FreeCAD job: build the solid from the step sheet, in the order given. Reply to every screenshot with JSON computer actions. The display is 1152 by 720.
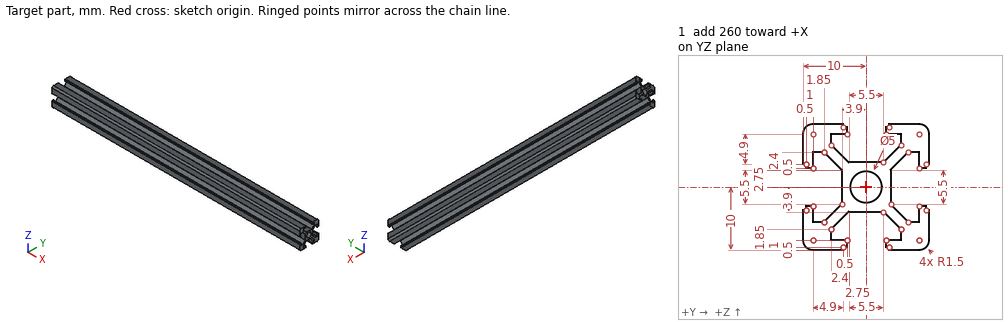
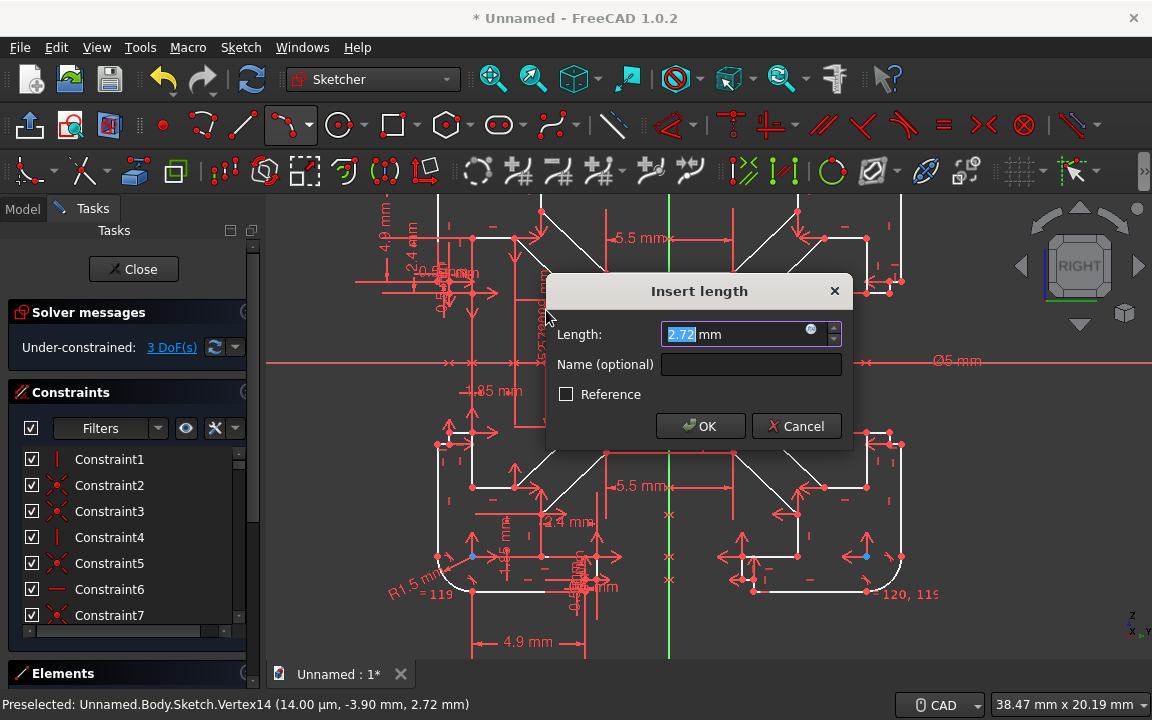
{"action": "type", "text": "2.75"}
{"action": "key", "text": "Return"}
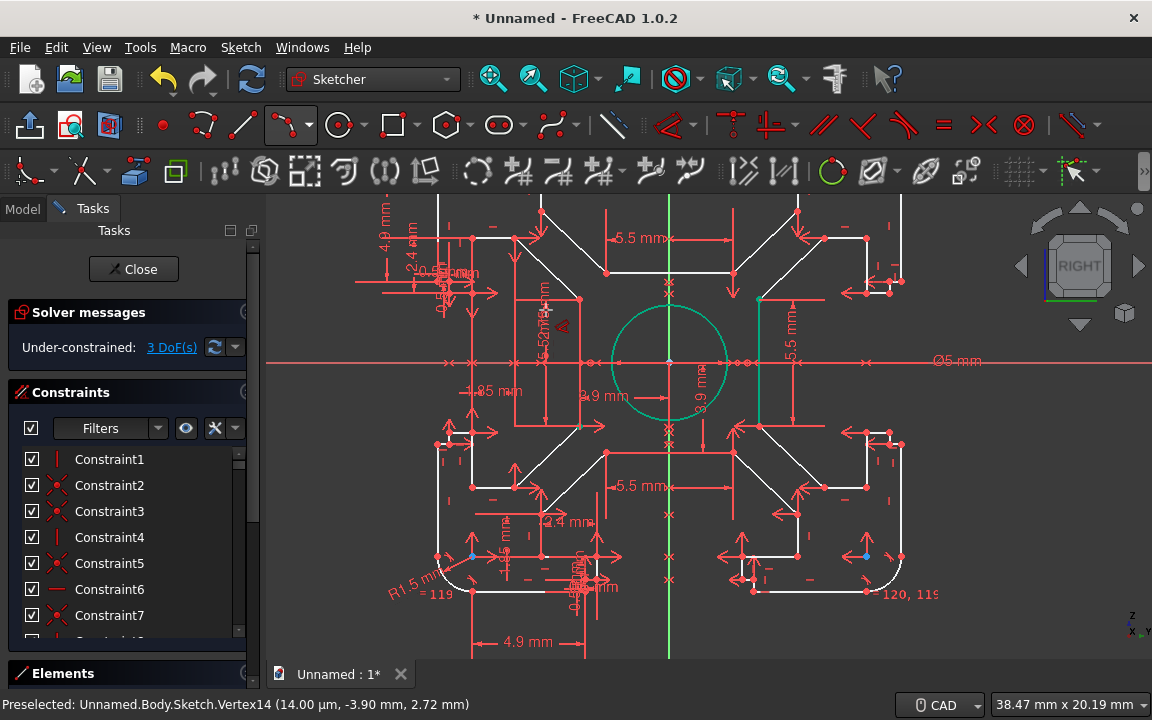
{"action": "left_click", "coordinate": [606, 453]}
{"action": "left_click", "coordinate": [652, 329]}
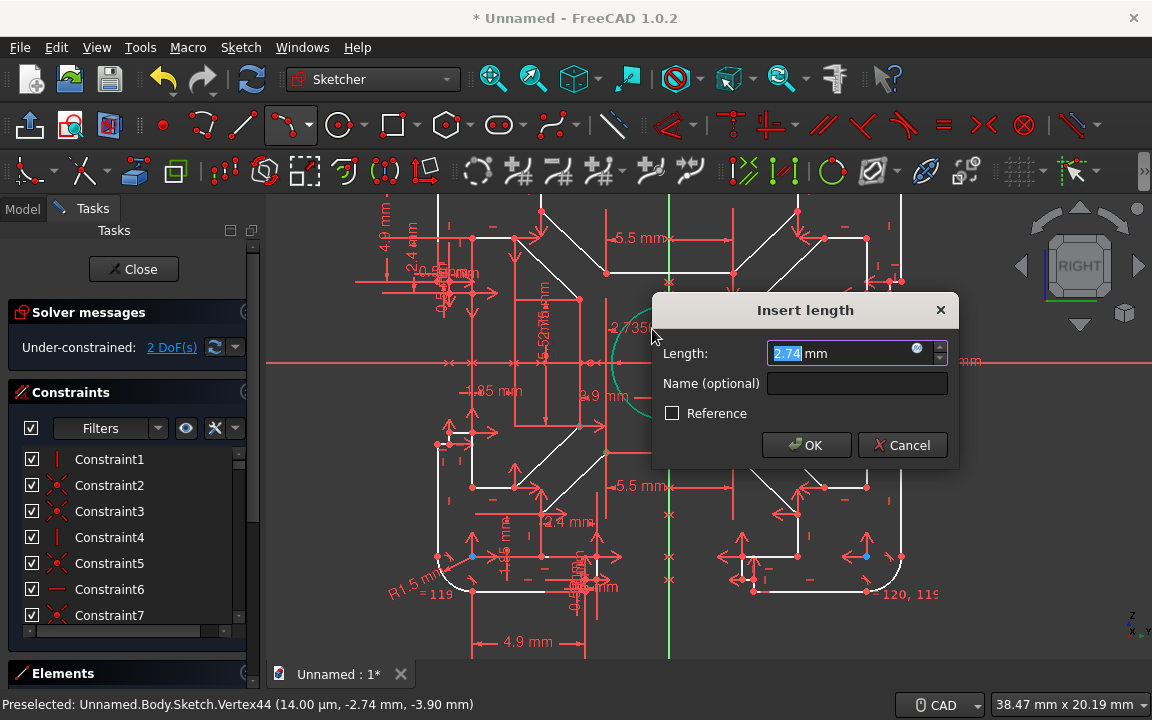
{"action": "type", "text": "2.75"}
{"action": "key", "text": "Return"}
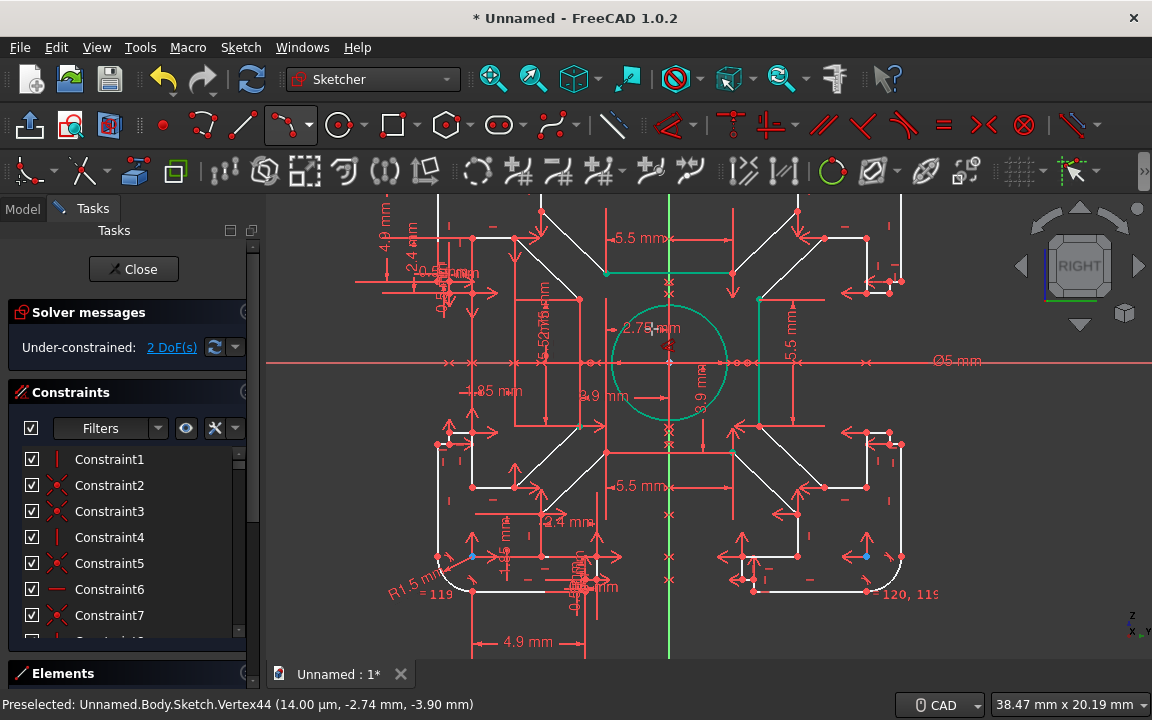
{"action": "scroll", "coordinate": [582, 556], "scroll_direction": "down", "scroll_amount": 2}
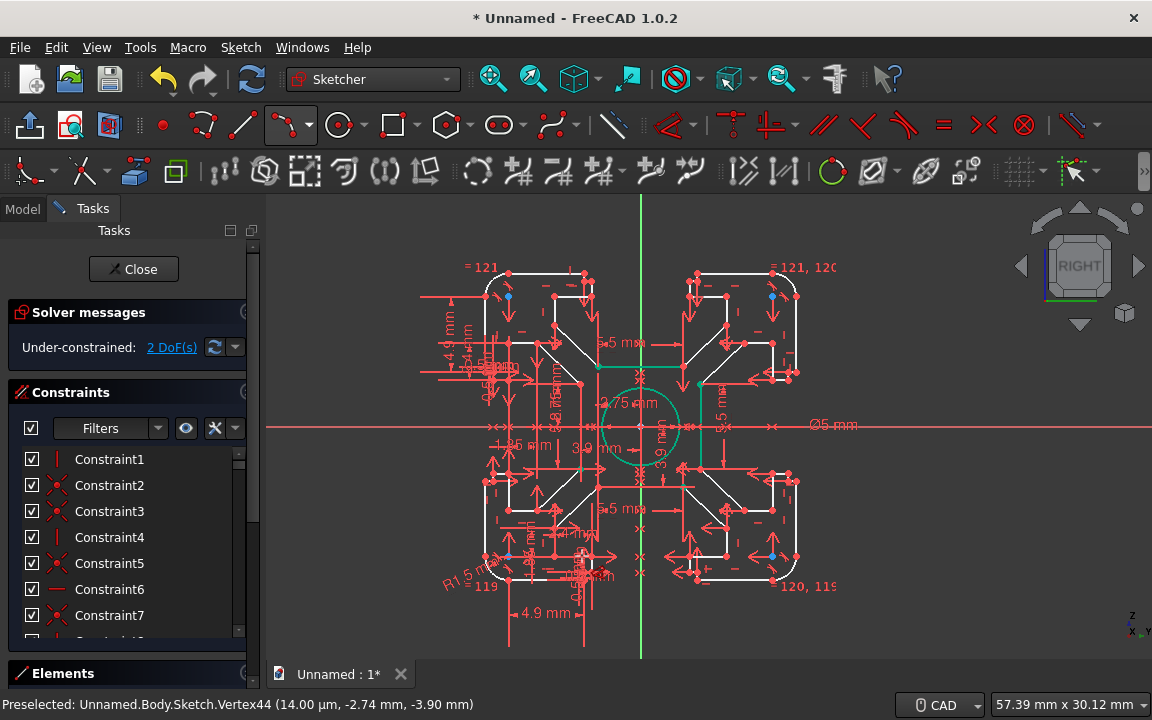
{"action": "left_click", "coordinate": [485, 297]}
{"action": "left_click", "coordinate": [599, 263]}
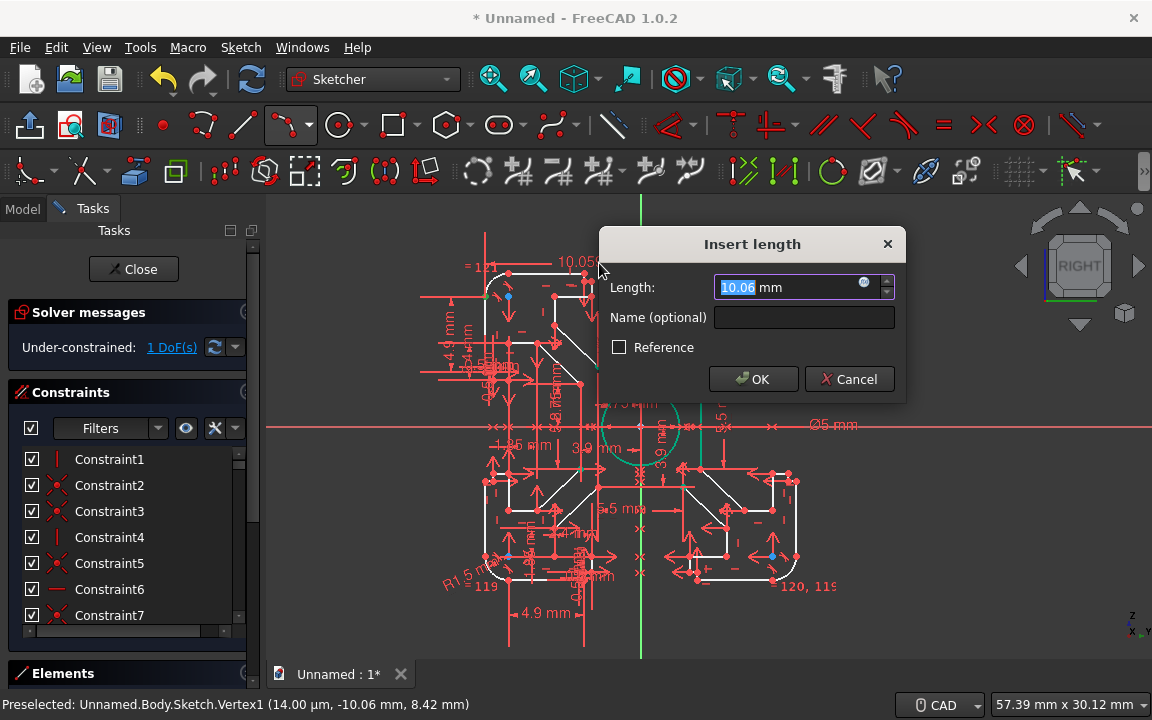
{"action": "type", "text": "10"}
{"action": "key", "text": "Return"}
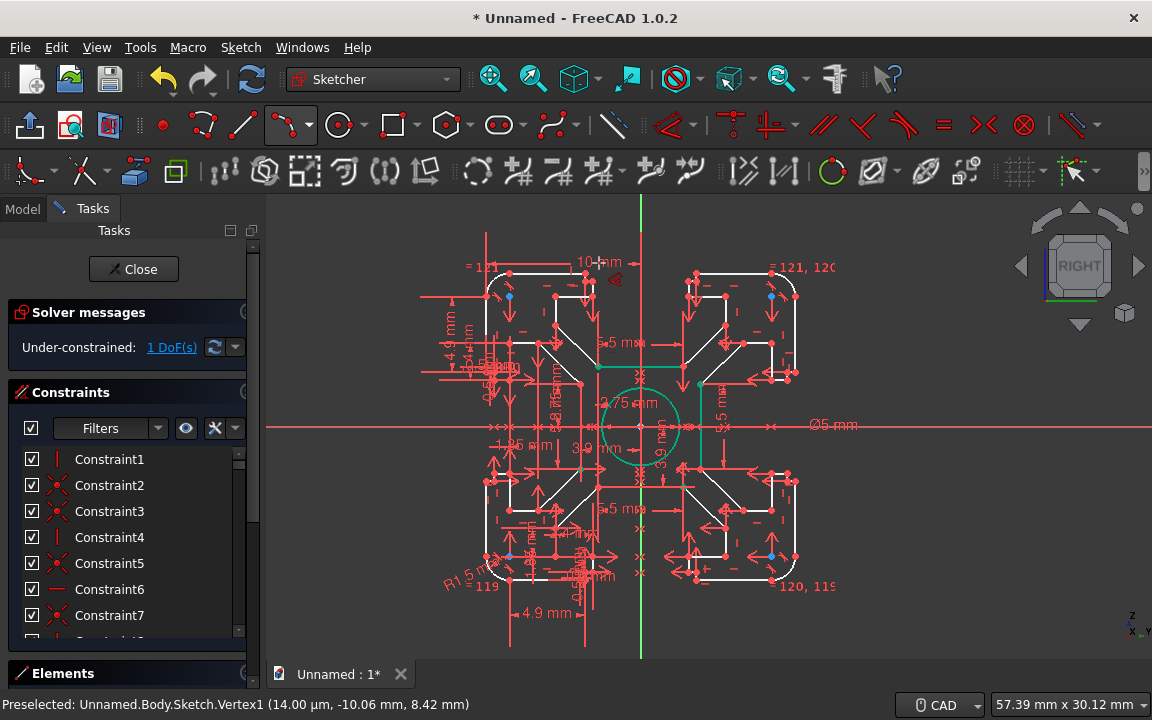
{"action": "left_click", "coordinate": [510, 580]}
{"action": "left_click", "coordinate": [476, 468]}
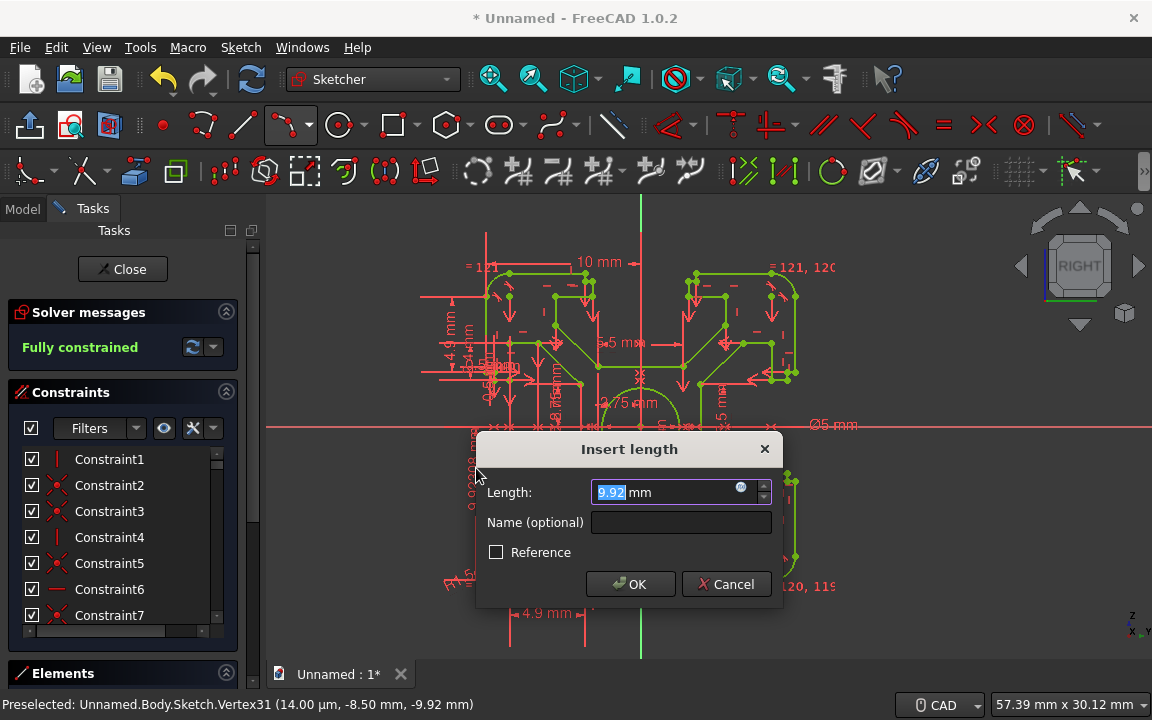
{"action": "type", "text": "10"}
{"action": "key", "text": "Return"}
{"action": "key", "text": "Escape"}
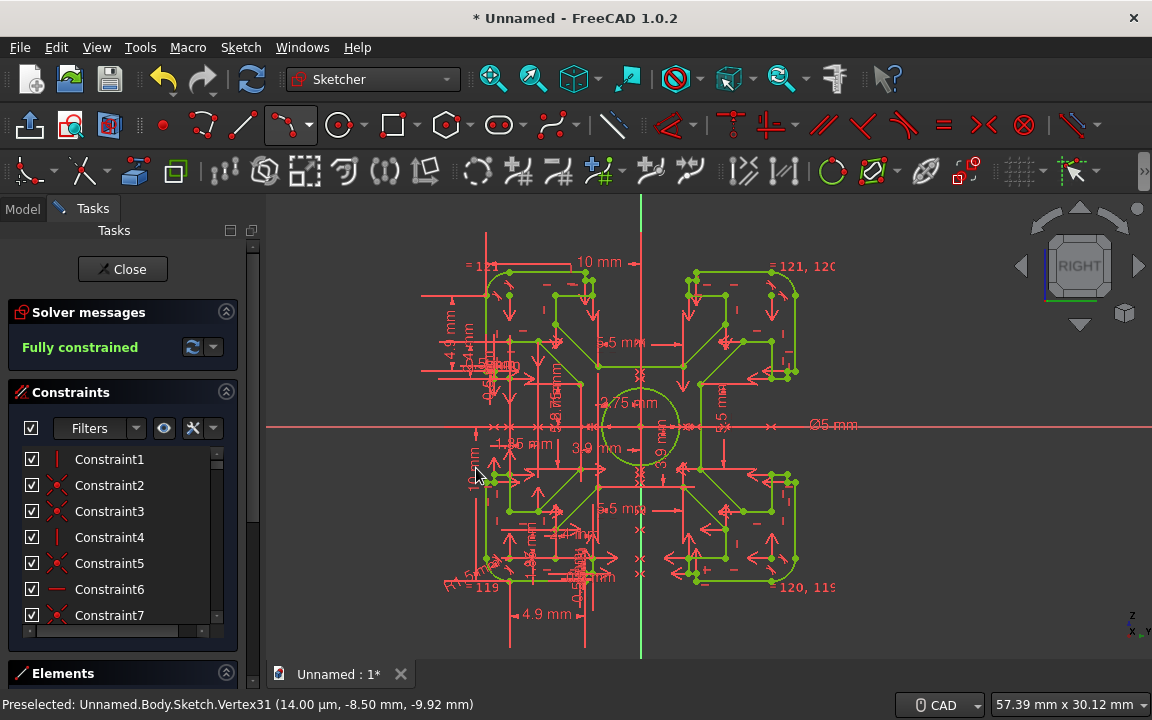
{"action": "left_click", "coordinate": [123, 269]}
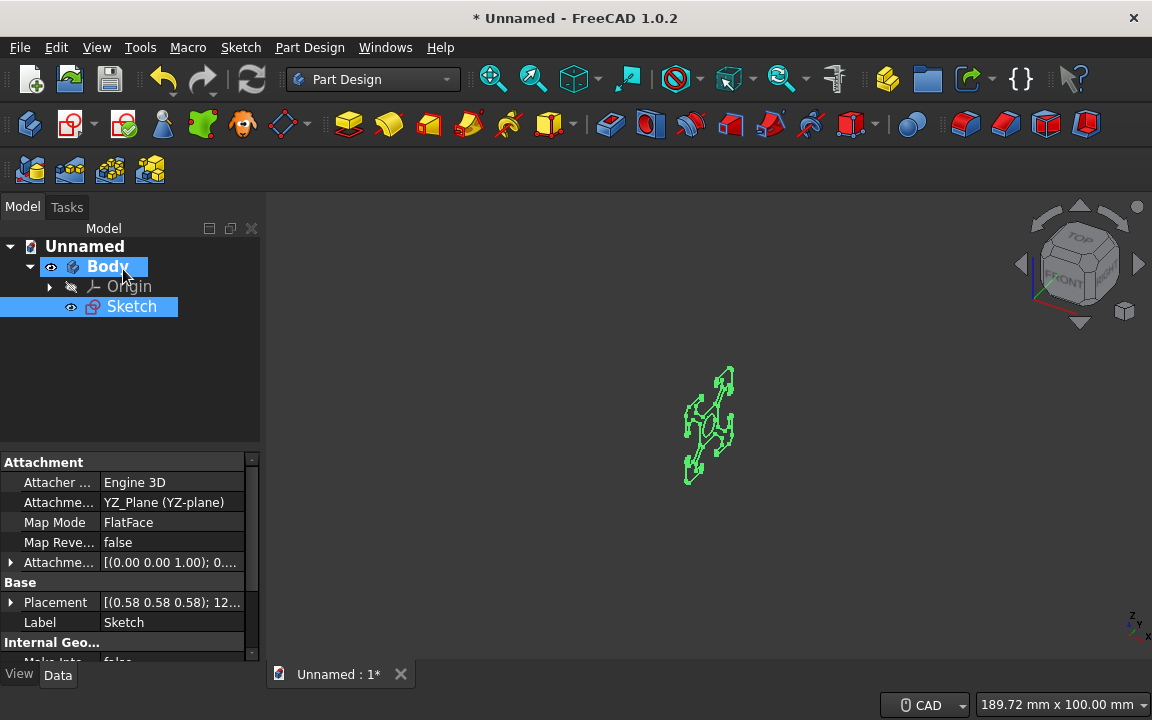
{"action": "left_click", "coordinate": [350, 124]}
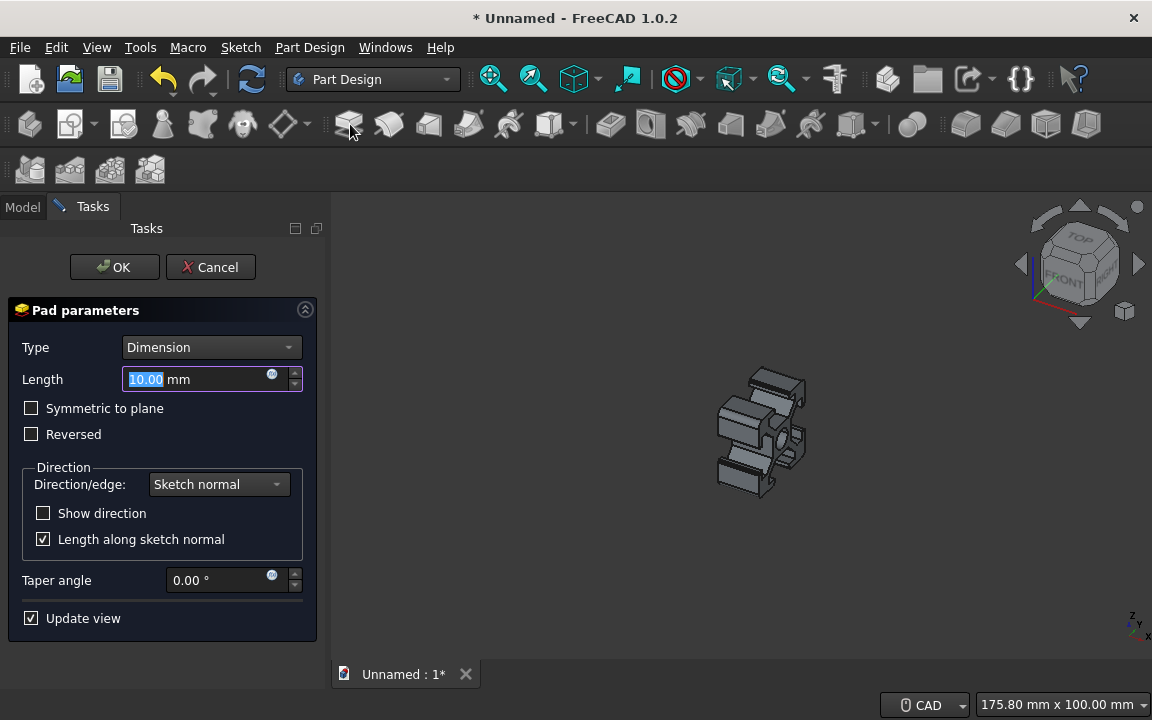
{"action": "type", "text": "260"}
{"action": "key", "text": "Tab"}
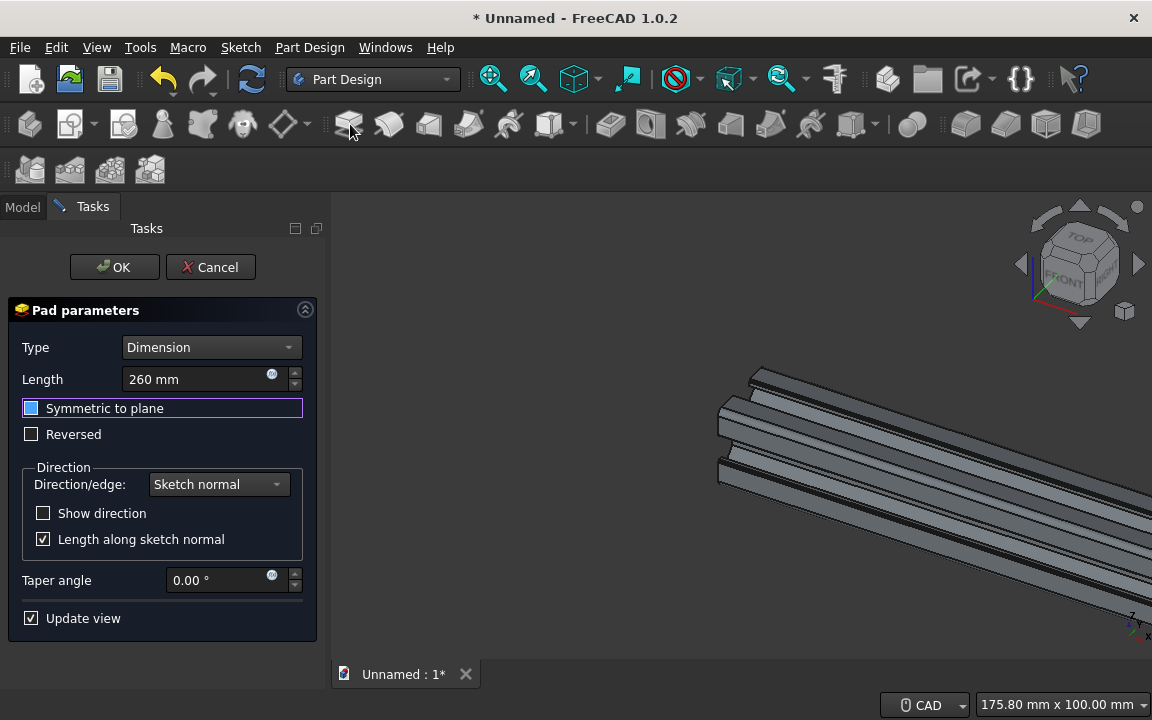
{"action": "left_click", "coordinate": [115, 267]}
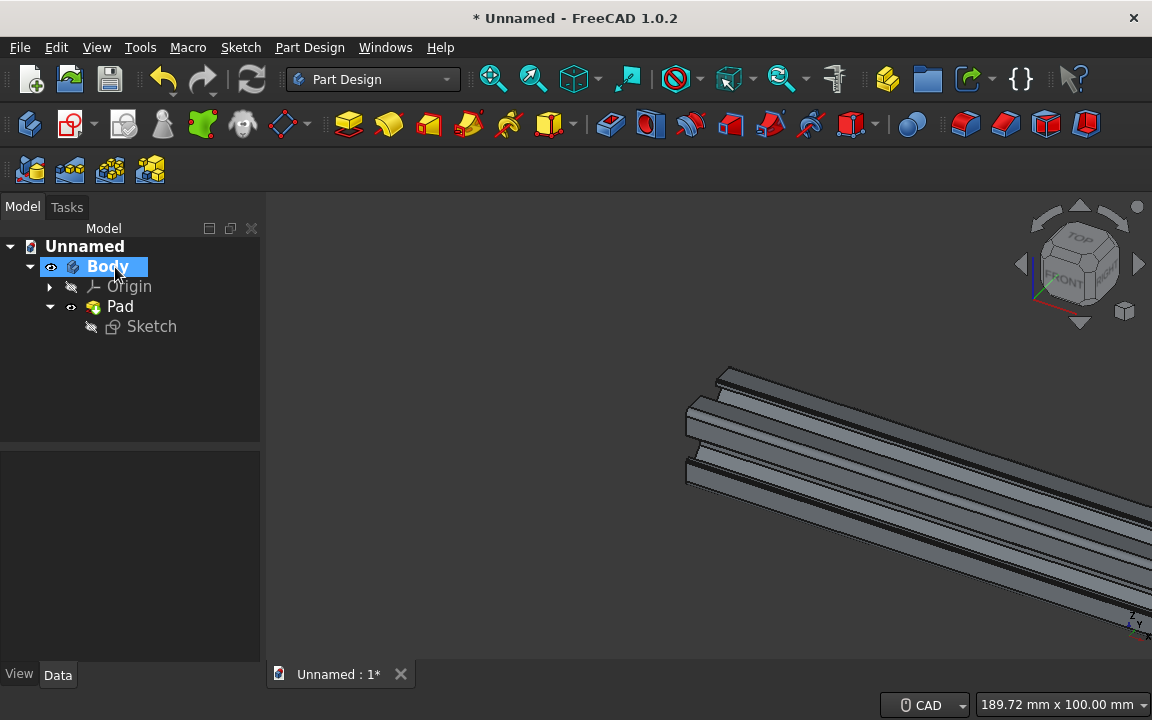
{"action": "key", "text": "0"}